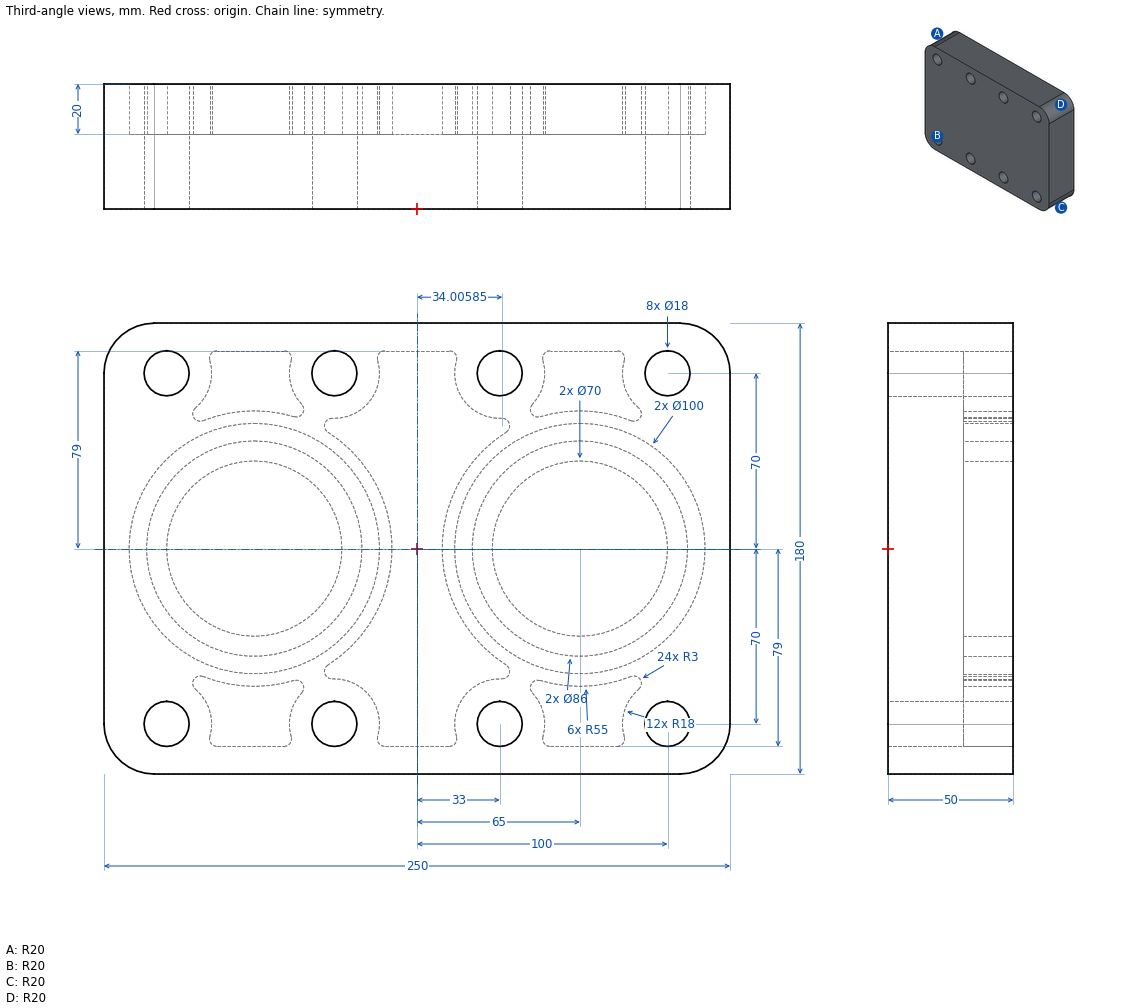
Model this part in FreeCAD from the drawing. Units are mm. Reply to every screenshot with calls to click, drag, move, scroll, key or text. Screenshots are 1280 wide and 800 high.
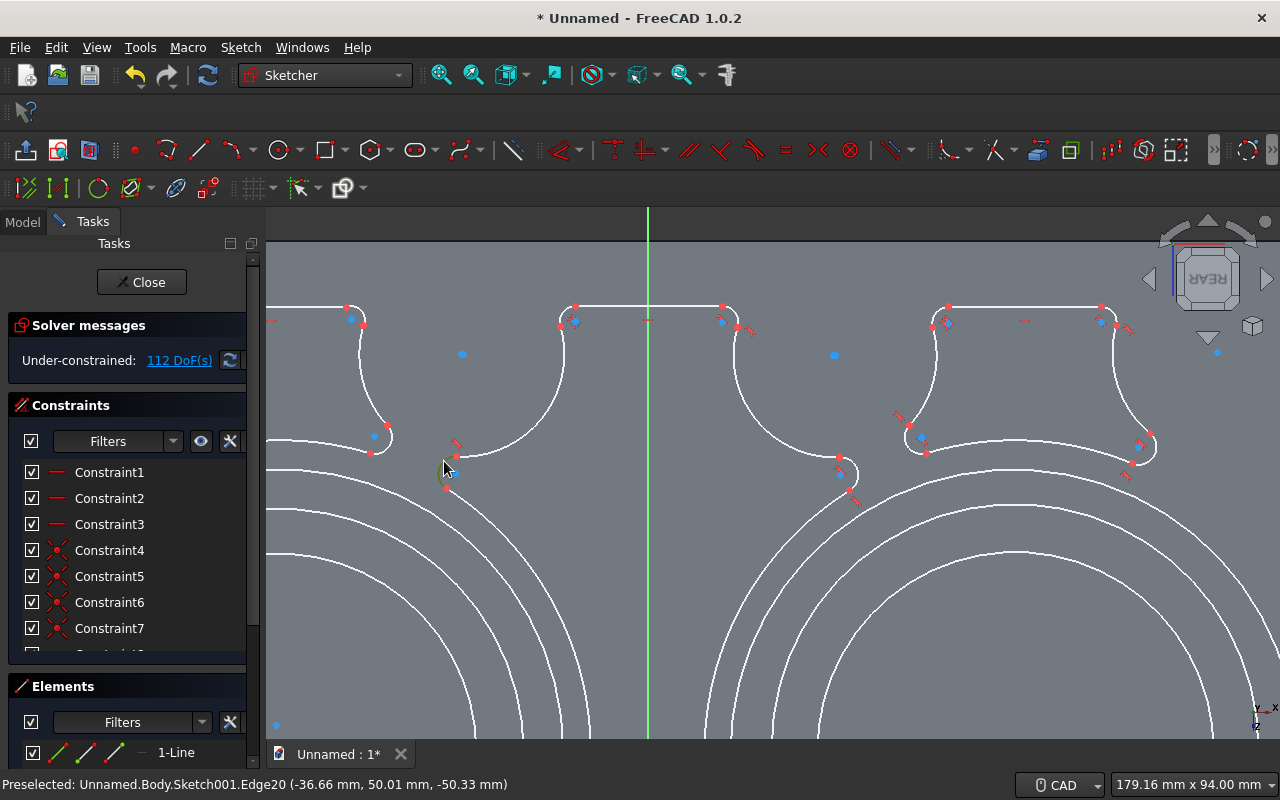
click(566, 630)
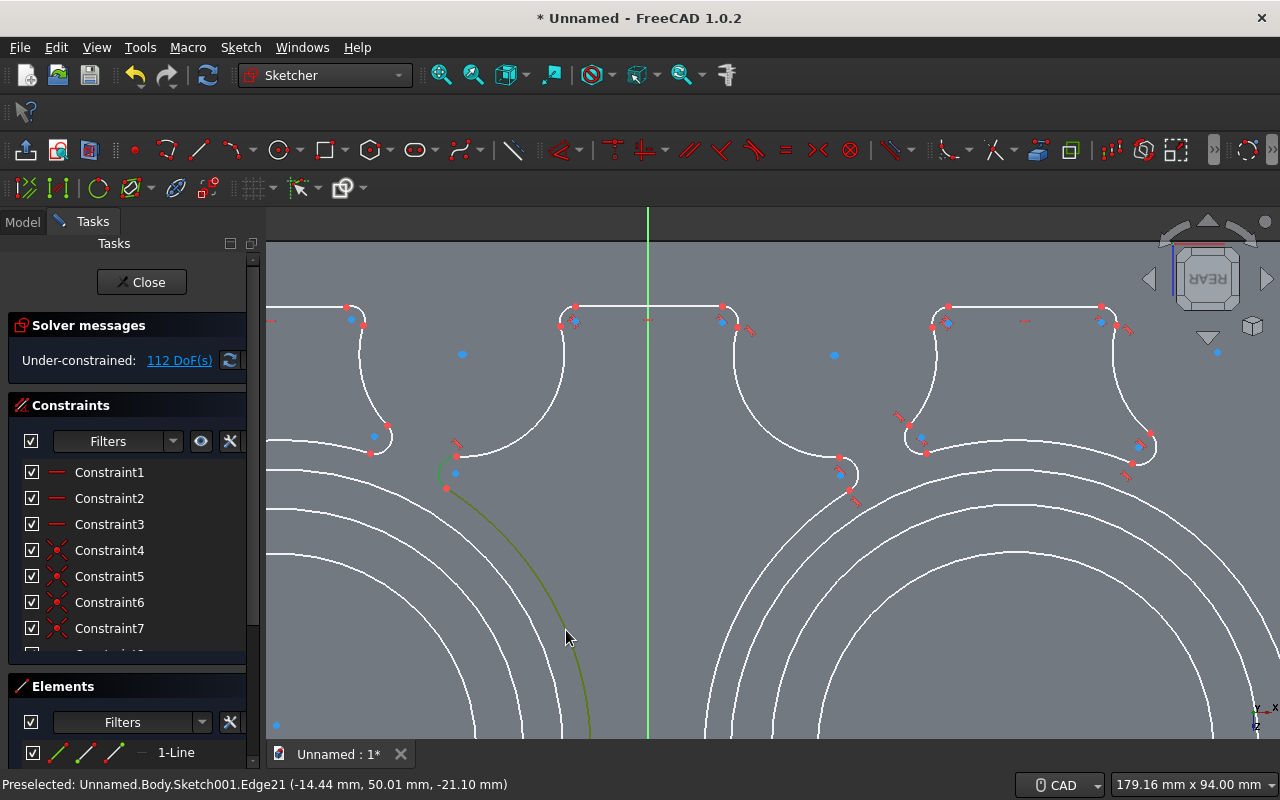
click(754, 150)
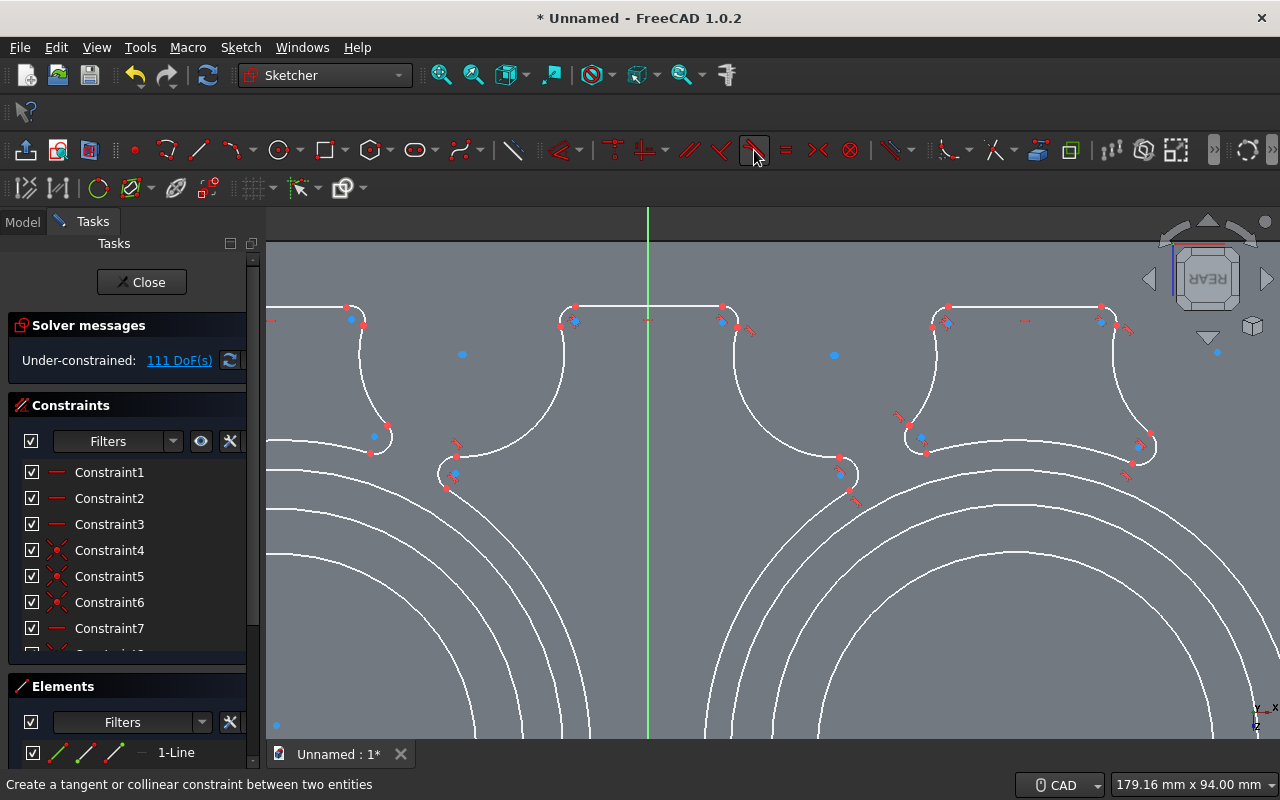
click(566, 630)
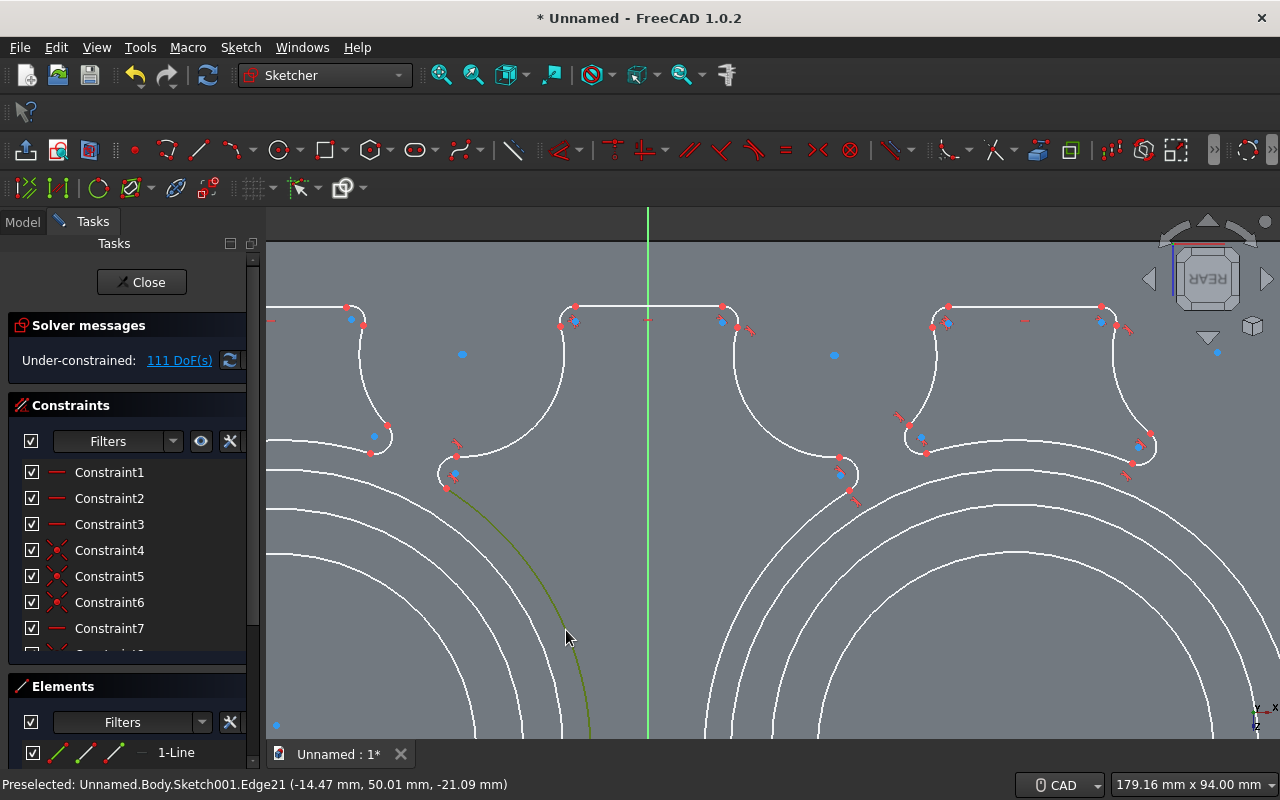
scroll(737, 312, down, 5)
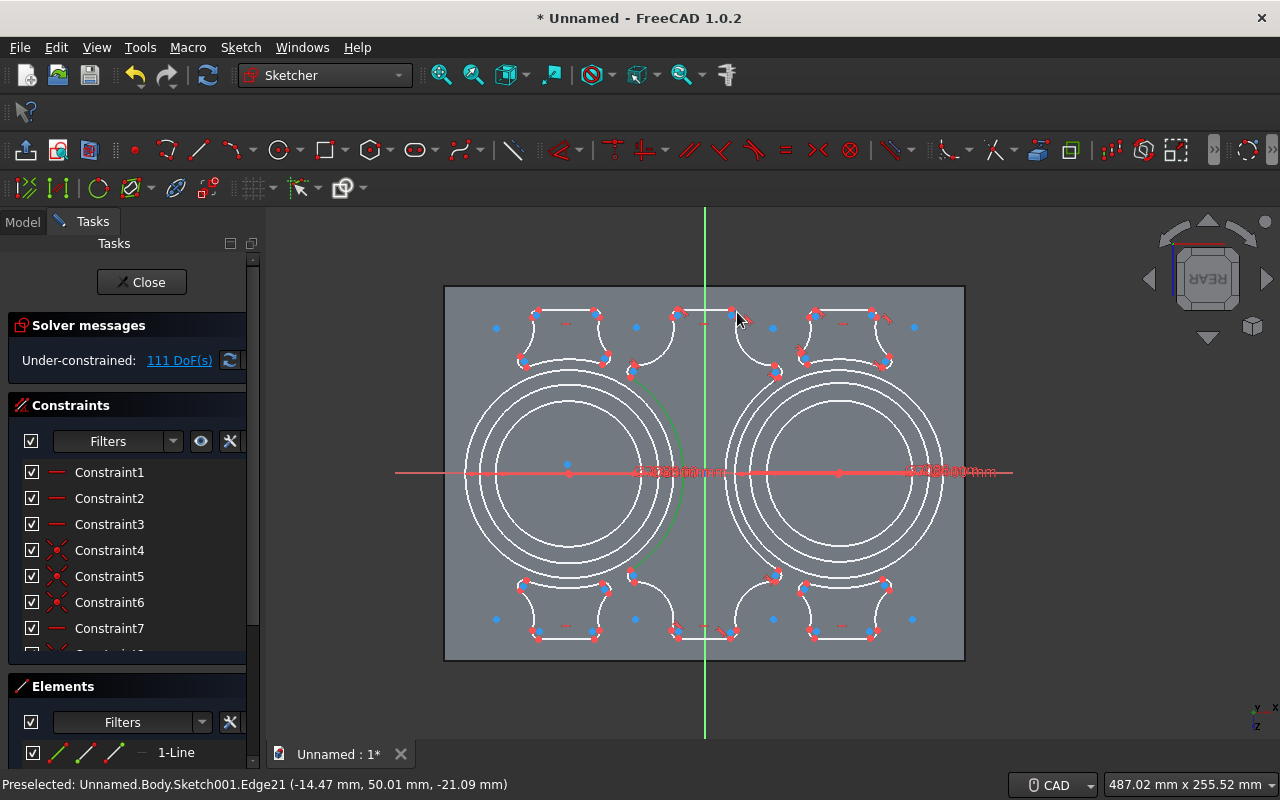
scroll(628, 575, up, 6)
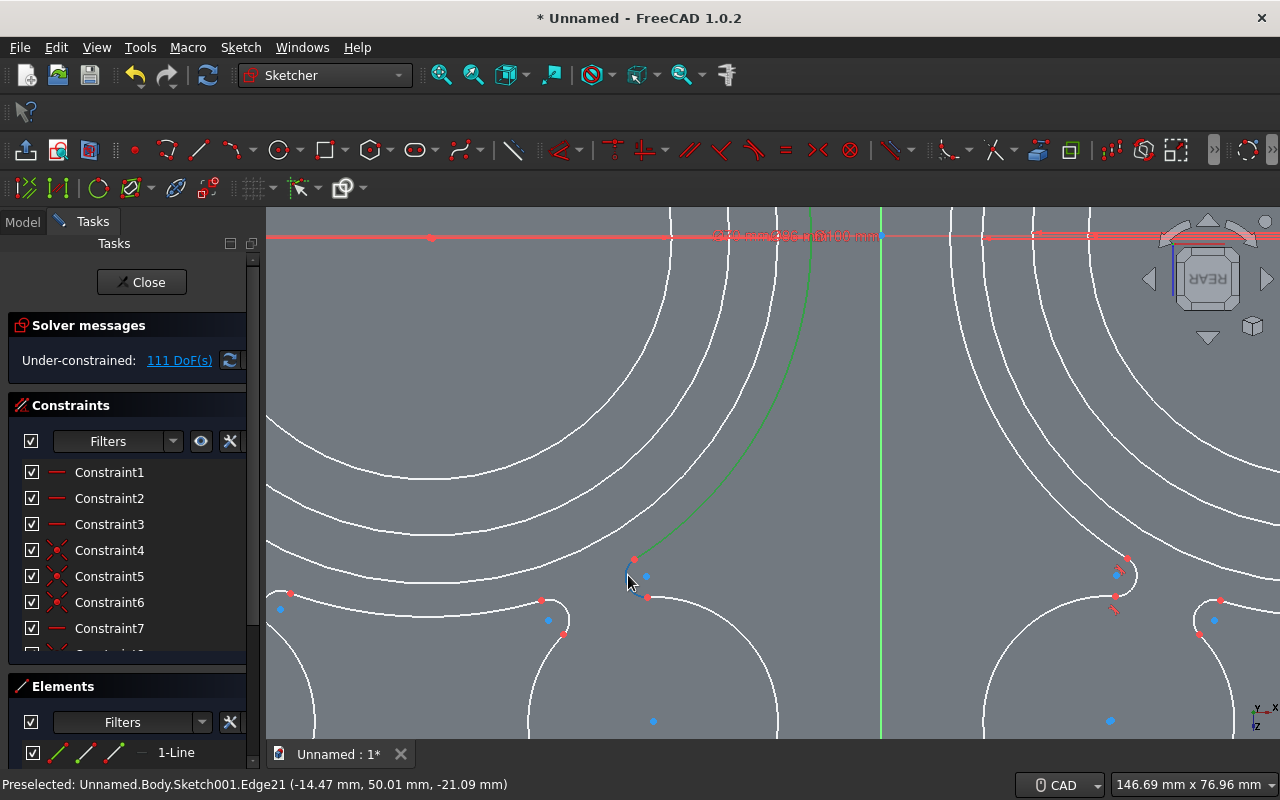
click(626, 573)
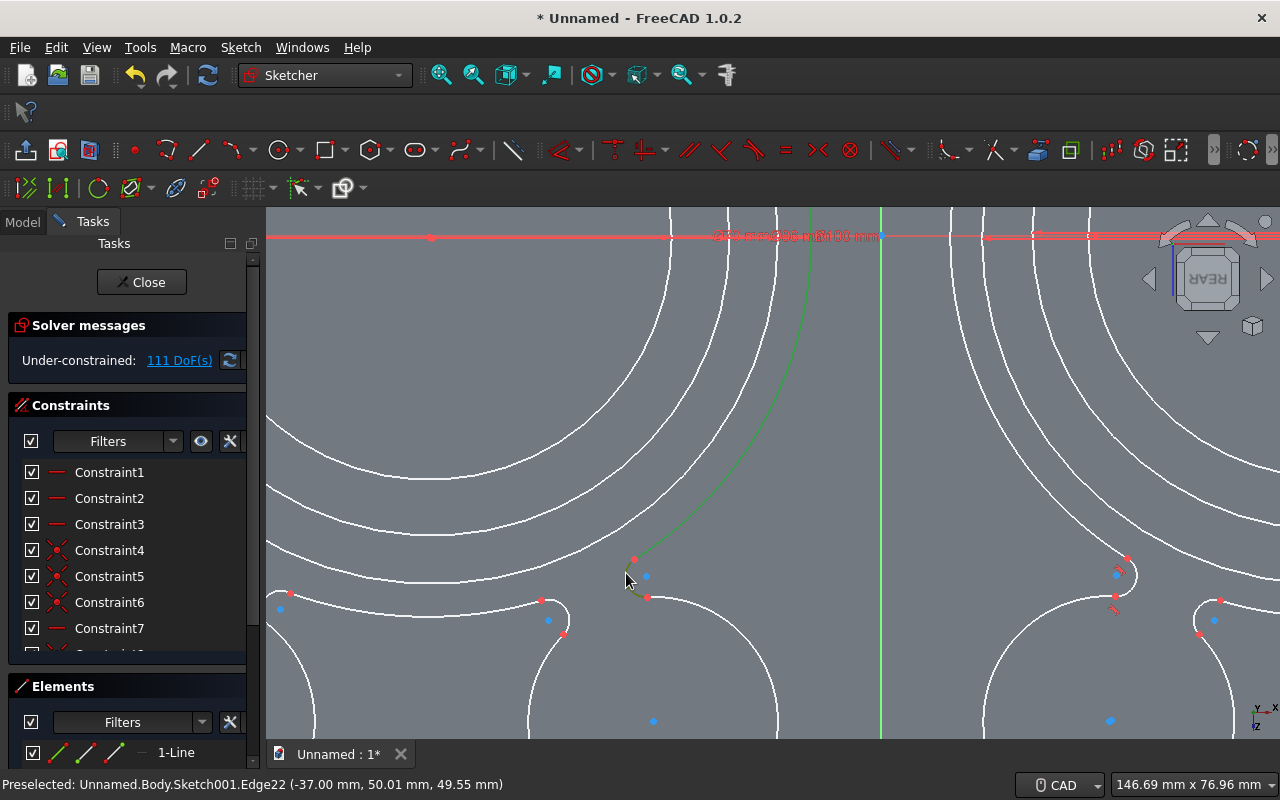
click(754, 150)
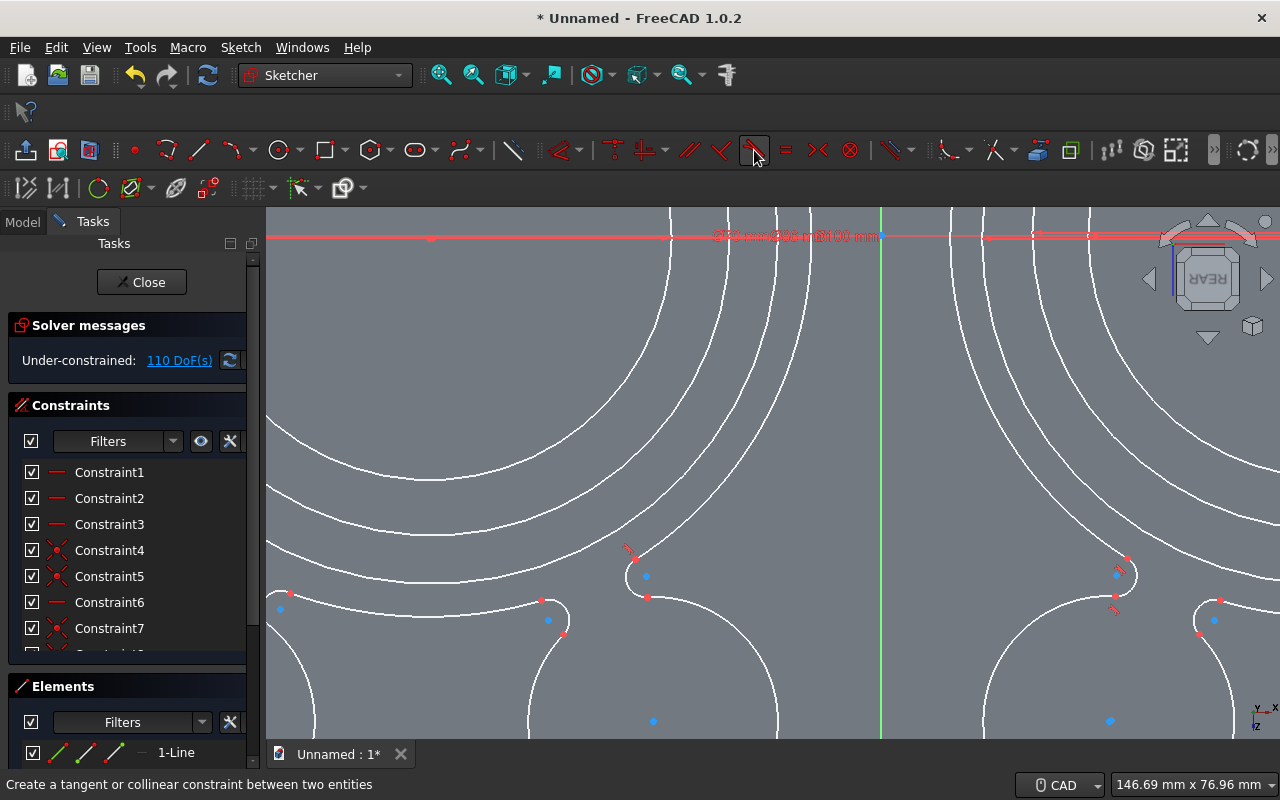
click(626, 573)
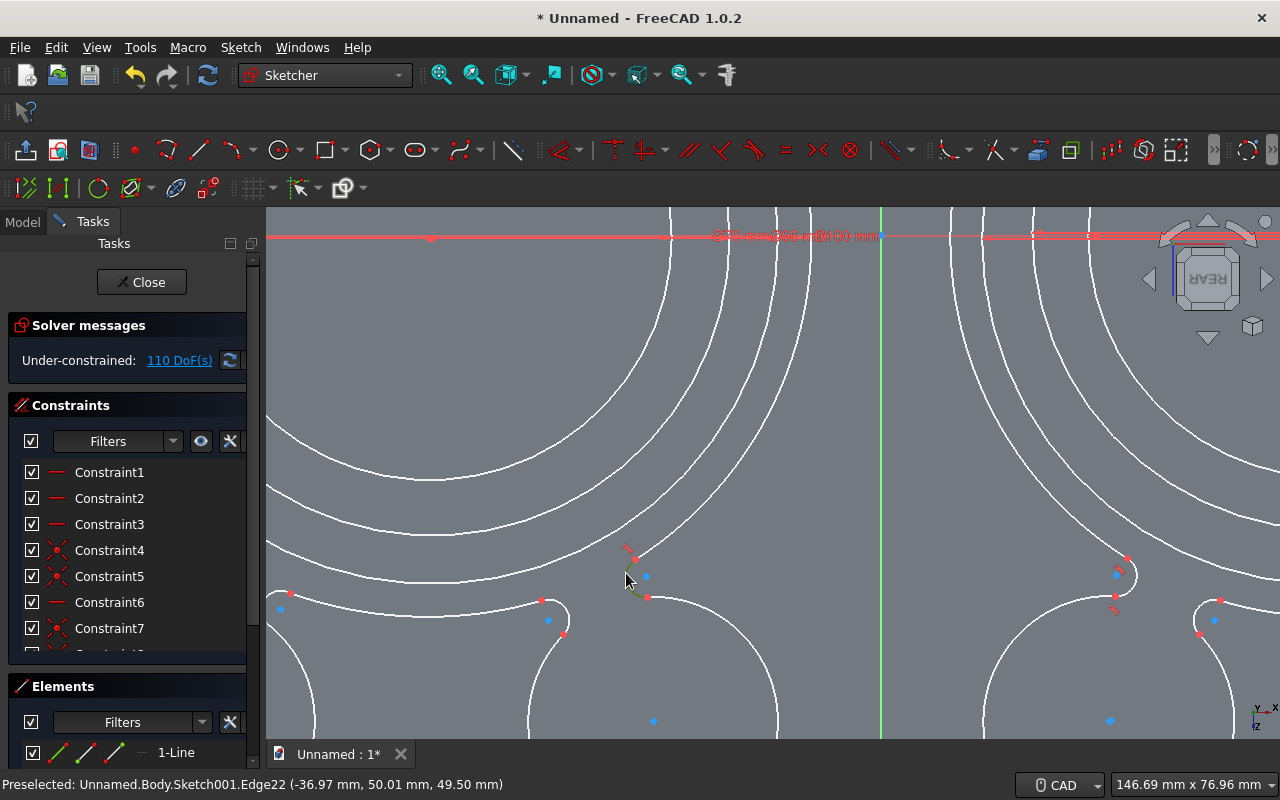
scroll(628, 575, down, 6)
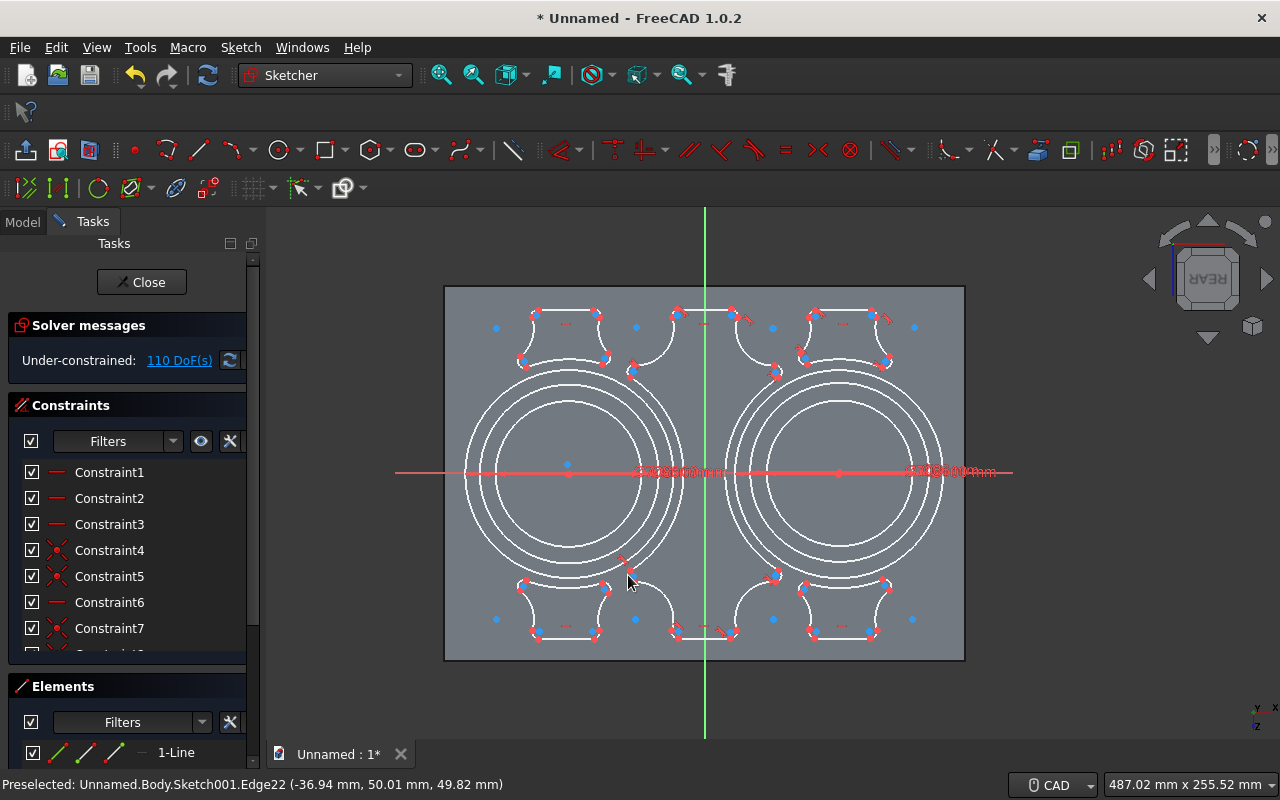
click(672, 609)